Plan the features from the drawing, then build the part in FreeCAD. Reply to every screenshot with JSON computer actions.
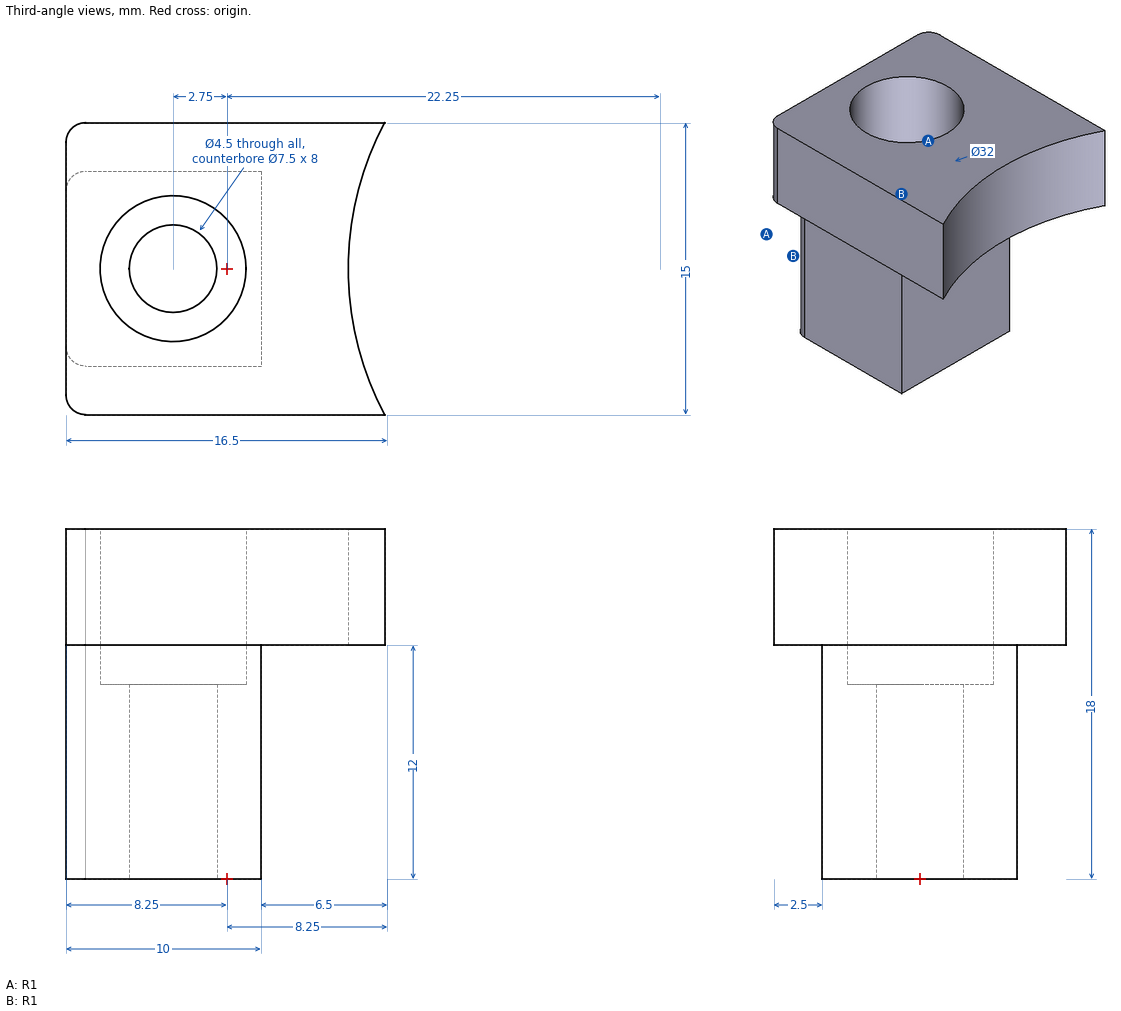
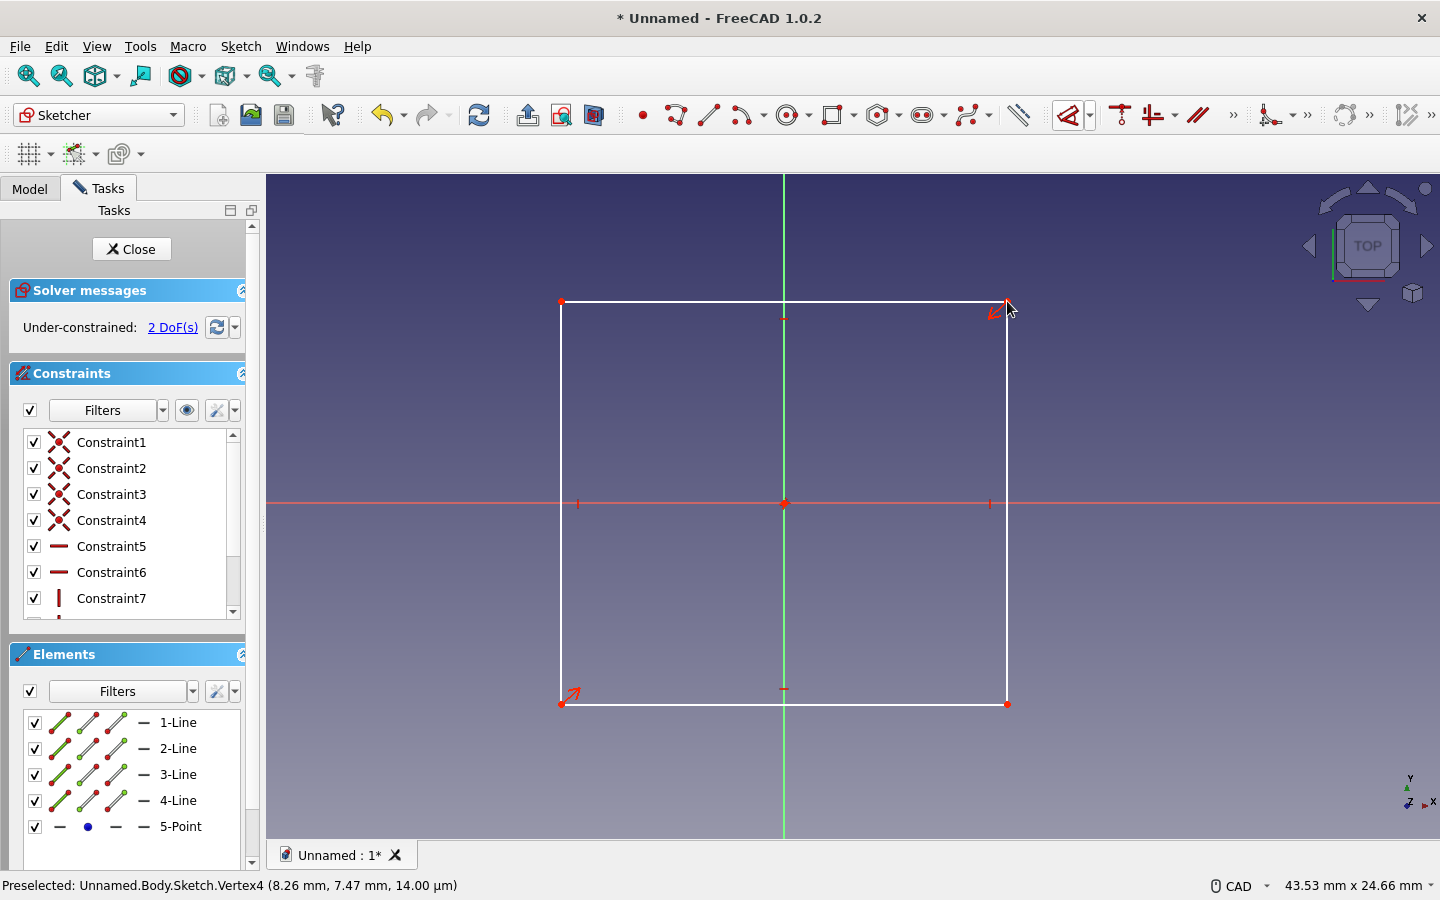
{"action": "left_click", "coordinate": [1068, 116]}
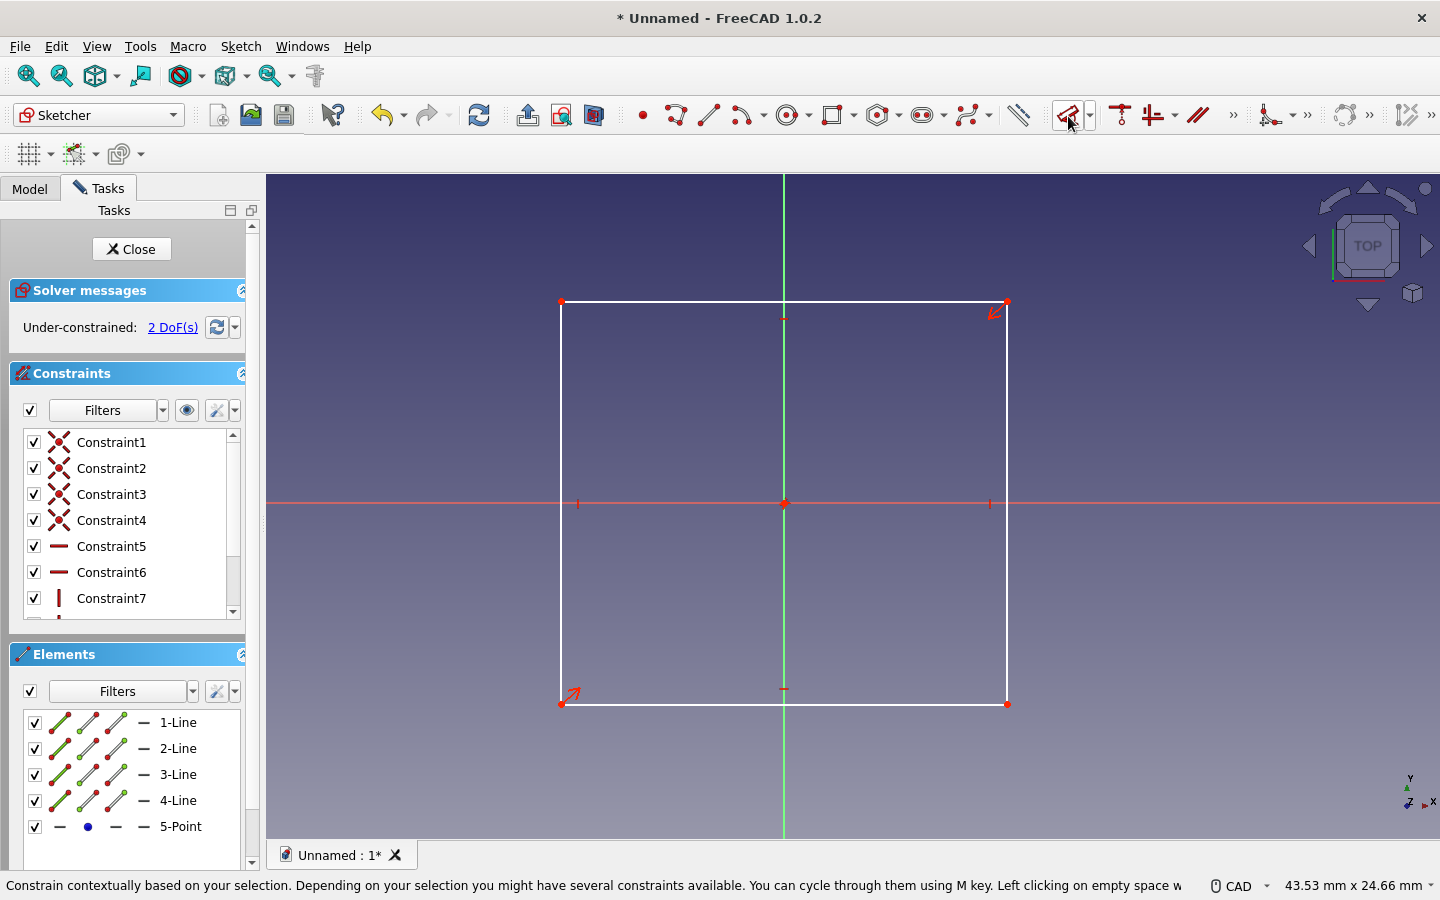
{"action": "left_click", "coordinate": [1007, 584]}
{"action": "left_click", "coordinate": [1041, 411]}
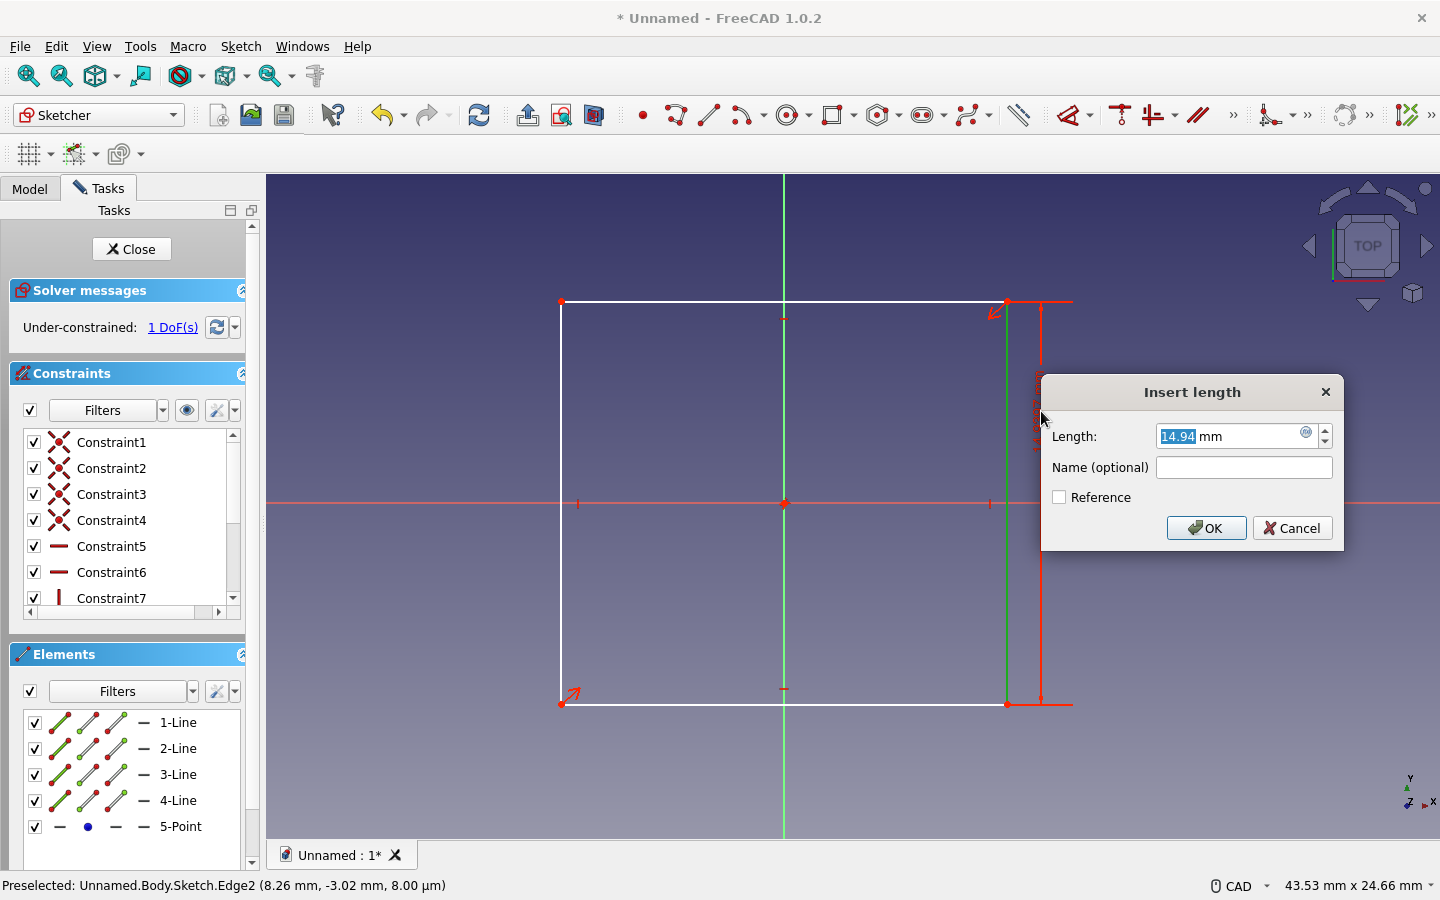
{"action": "type", "text": "15"}
{"action": "key", "text": "Return"}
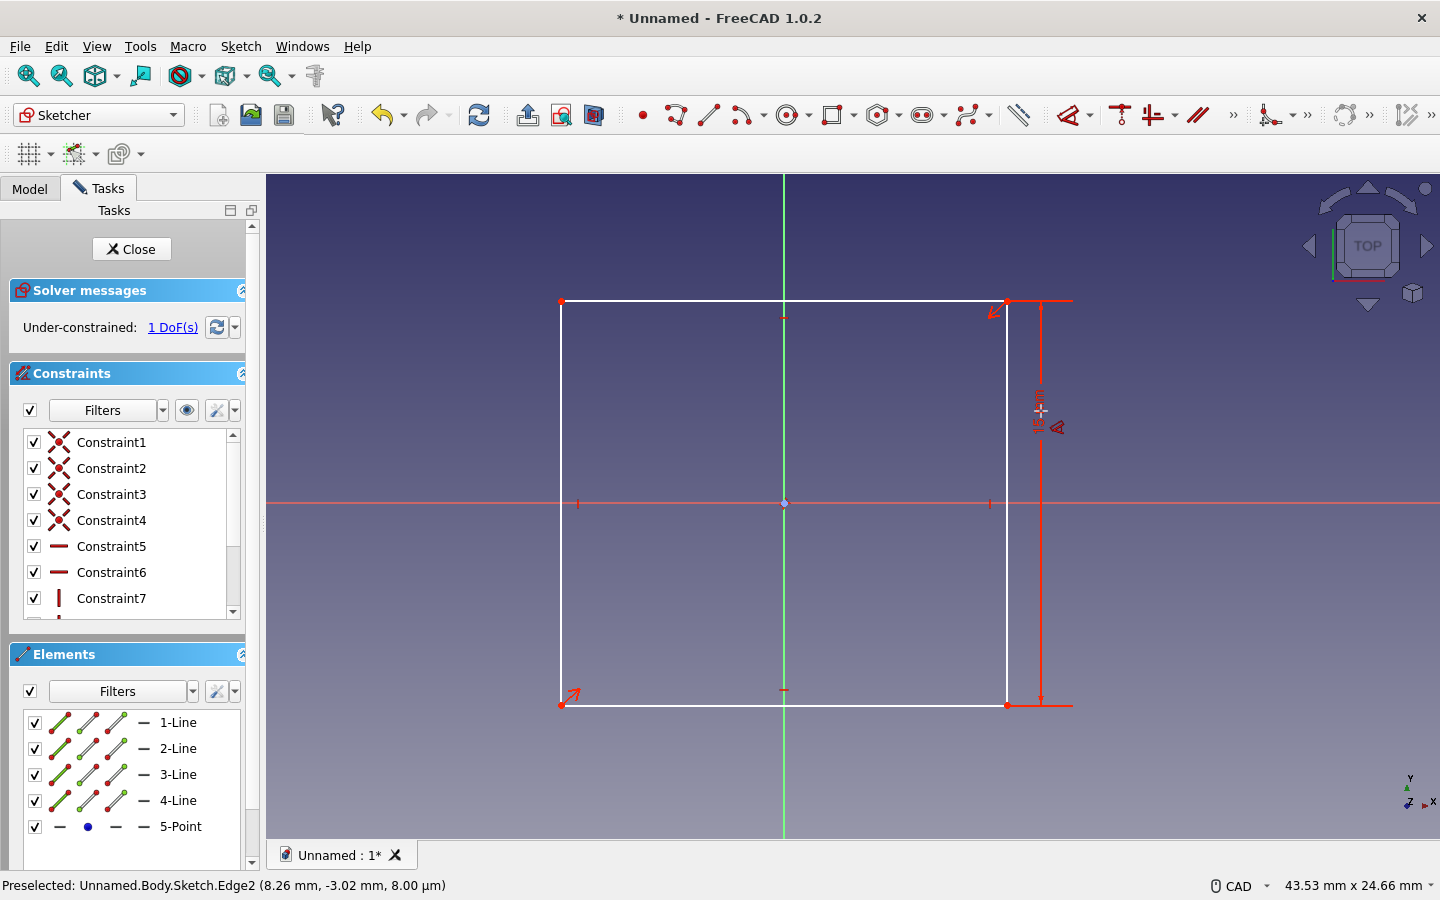
{"action": "left_click", "coordinate": [695, 706]}
{"action": "left_click", "coordinate": [682, 740]}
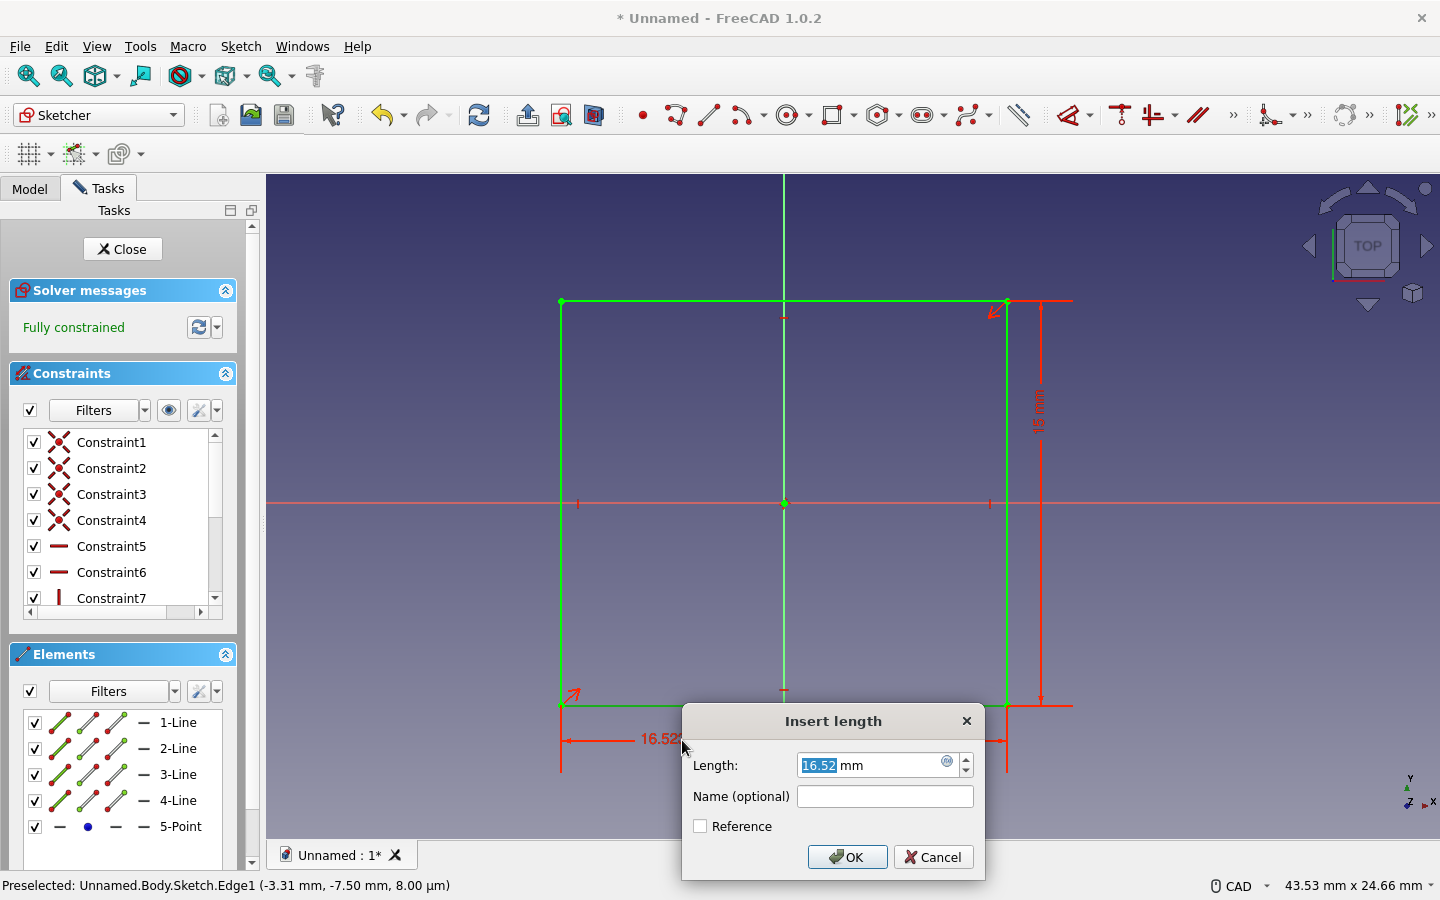
{"action": "type", "text": "16.5"}
{"action": "key", "text": "Return"}
{"action": "key", "text": "Escape"}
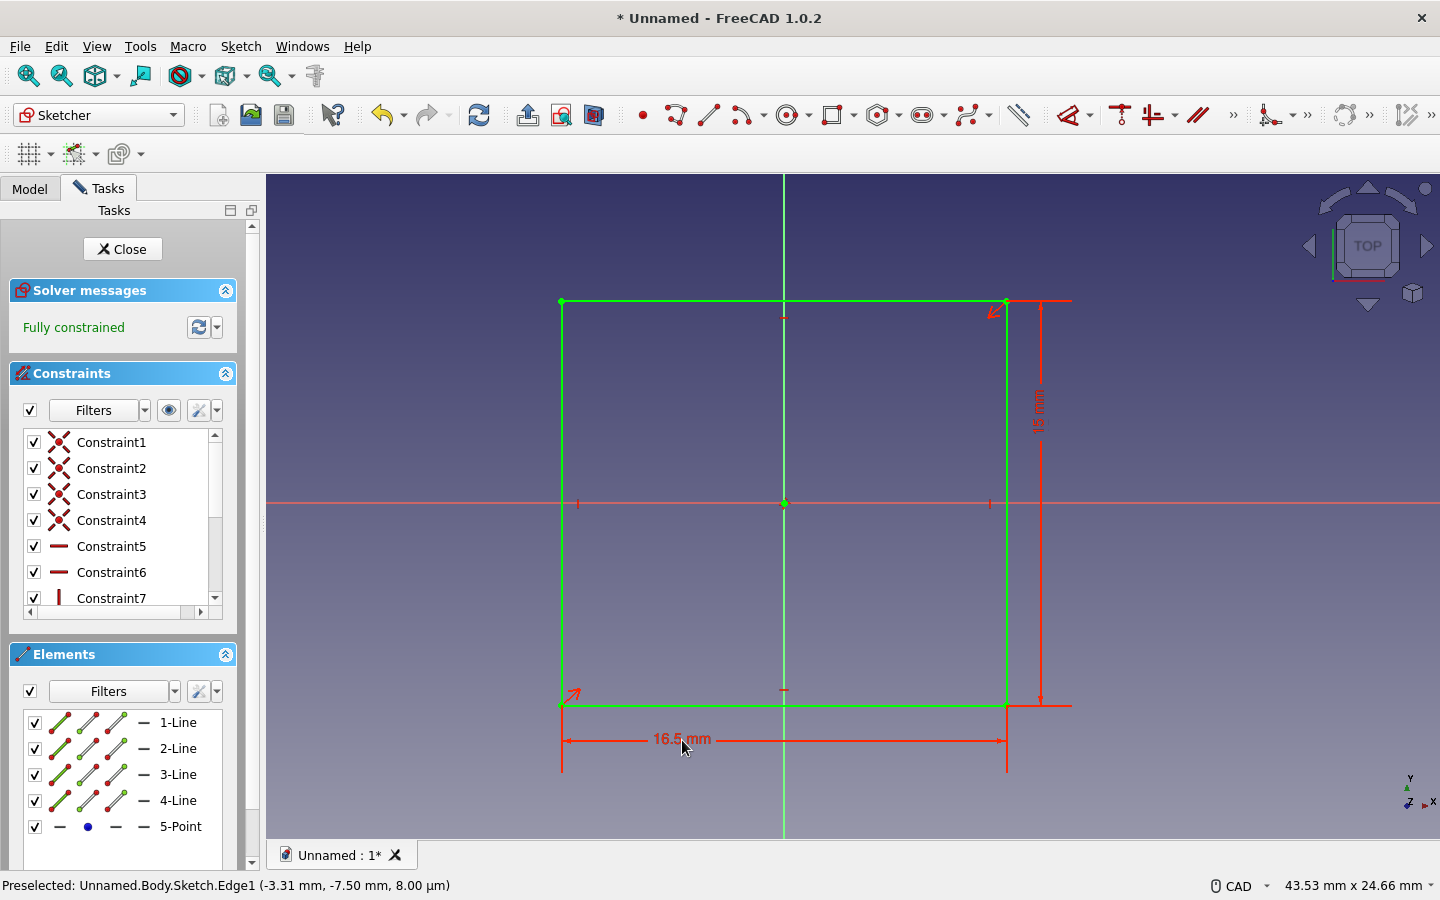
{"action": "left_click", "coordinate": [123, 249]}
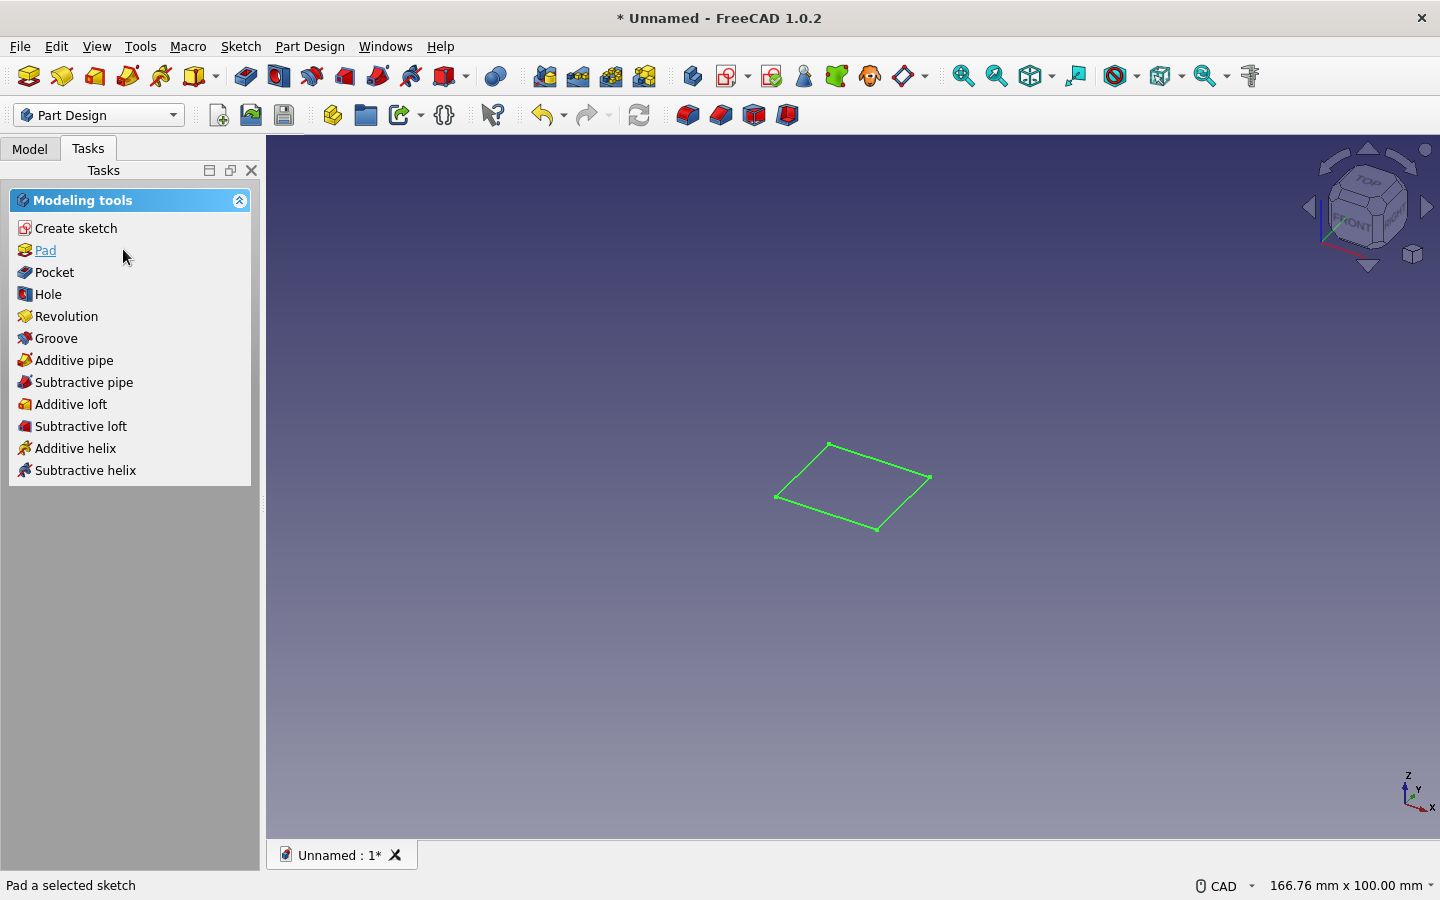
{"action": "left_click", "coordinate": [29, 76]}